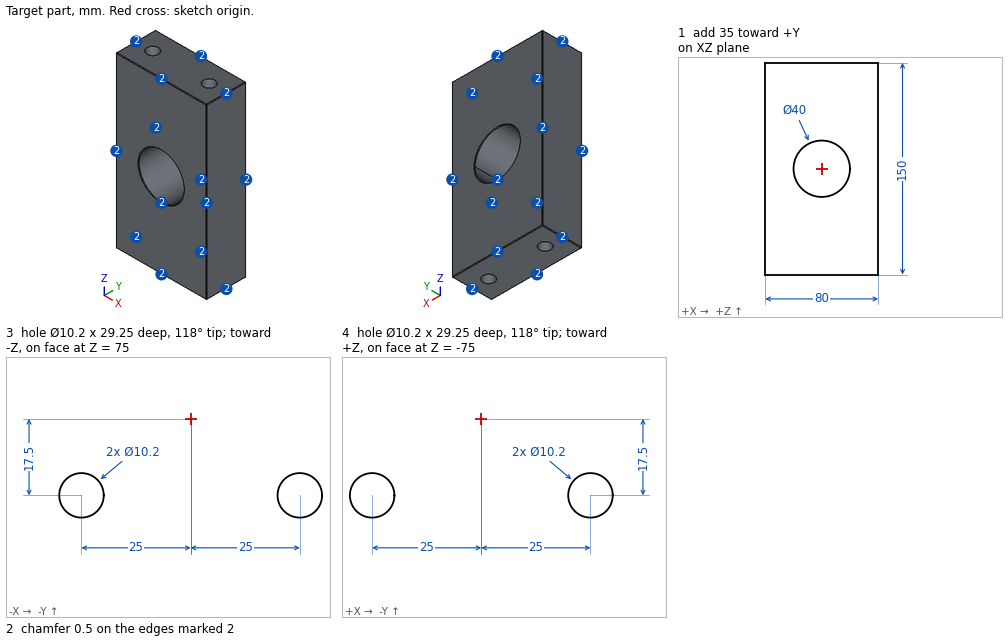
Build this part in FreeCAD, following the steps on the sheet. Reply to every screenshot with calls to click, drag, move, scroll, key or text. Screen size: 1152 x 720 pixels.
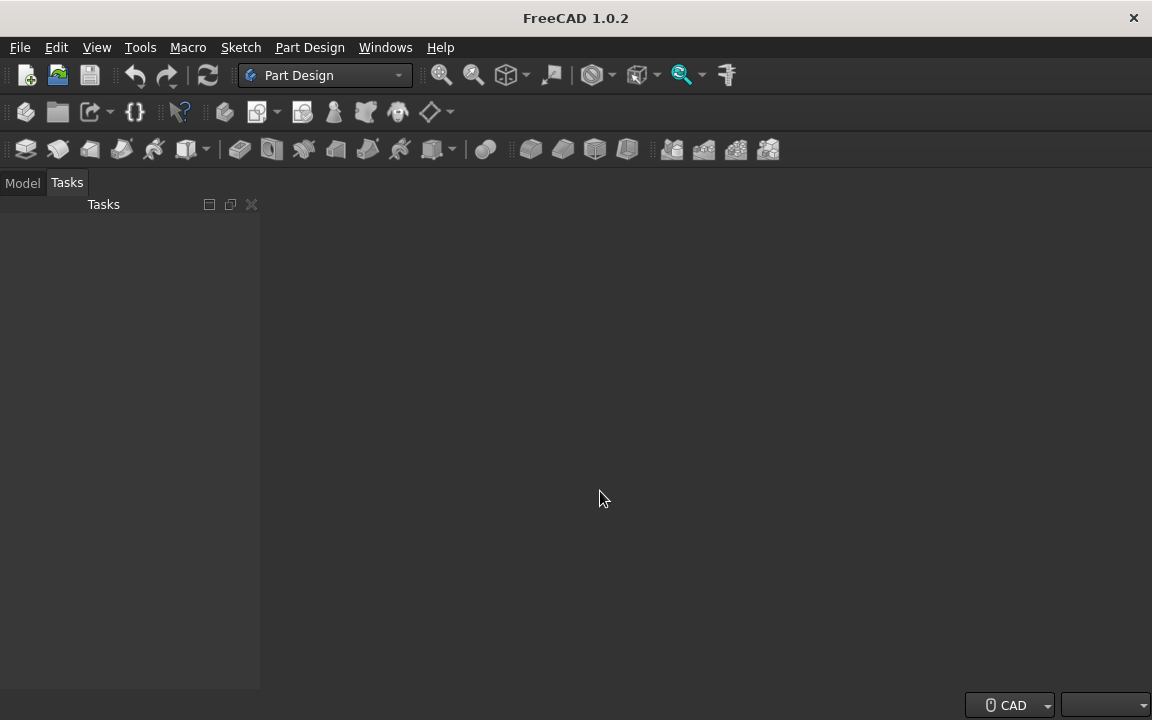
key(ctrl+n)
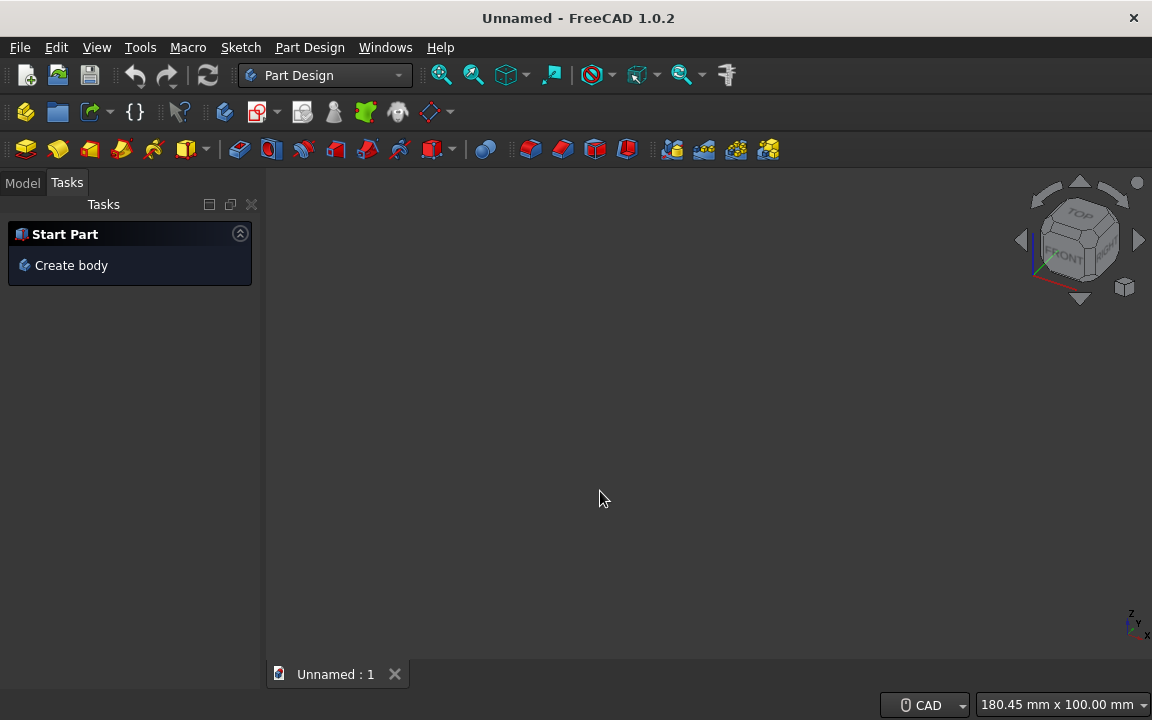
click(258, 112)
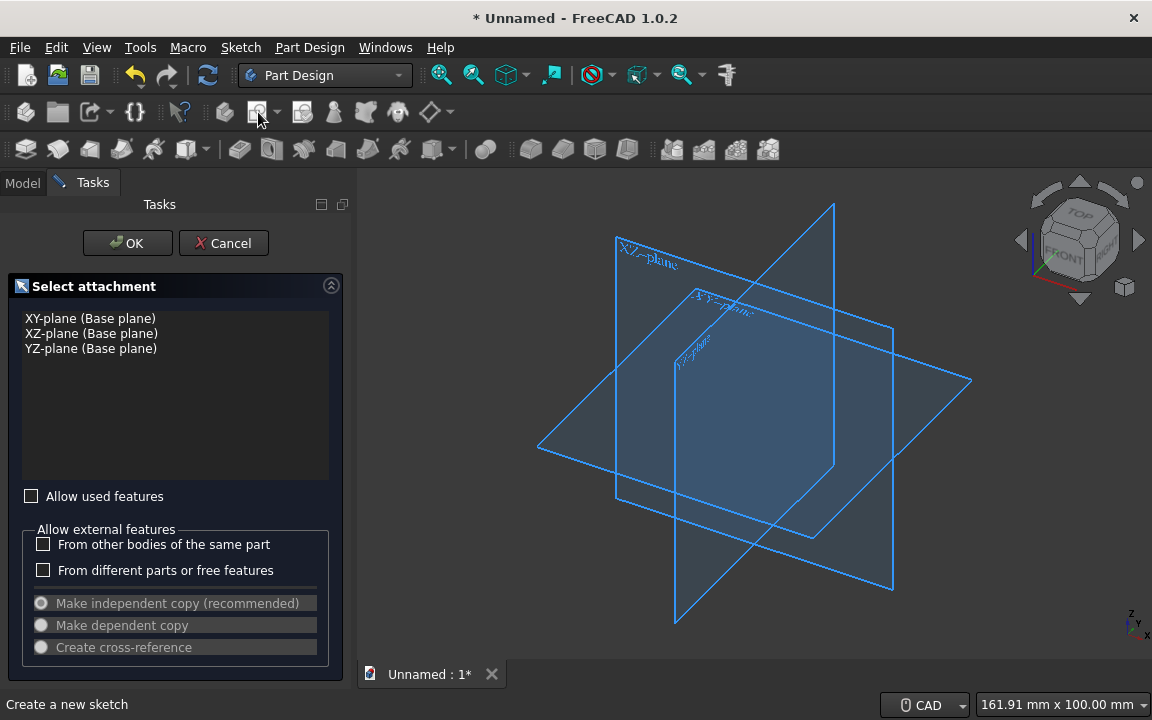
click(82, 334)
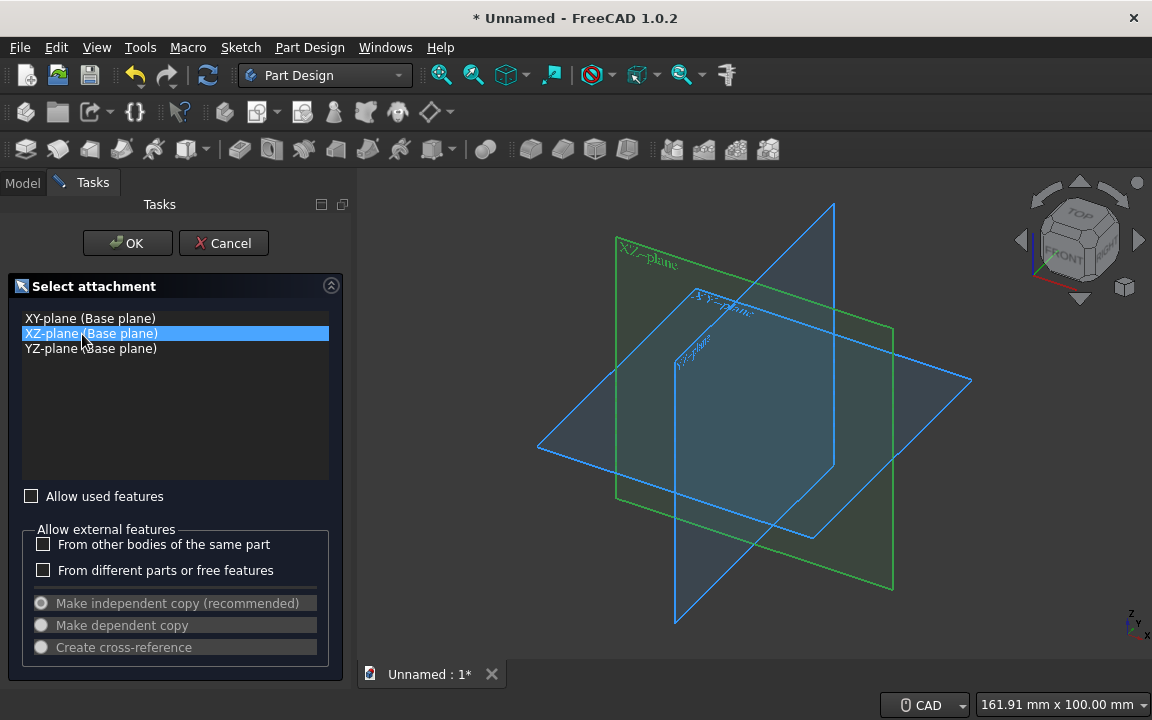
click(128, 243)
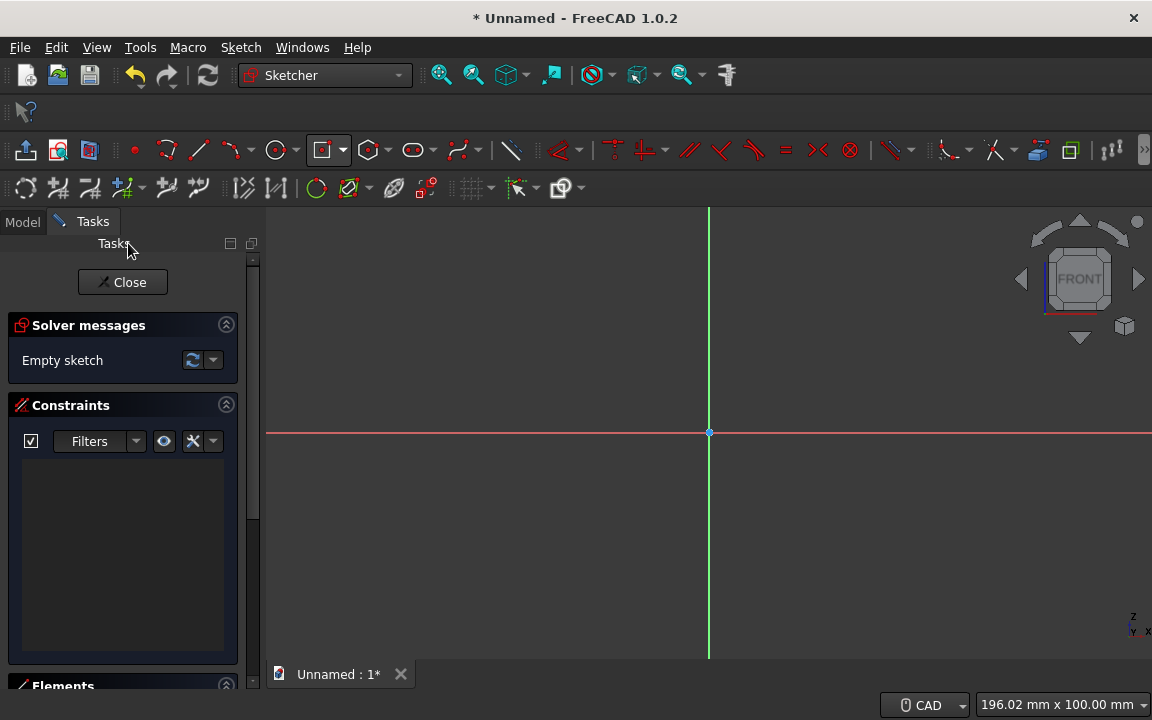
scroll(585, 433, down, 4)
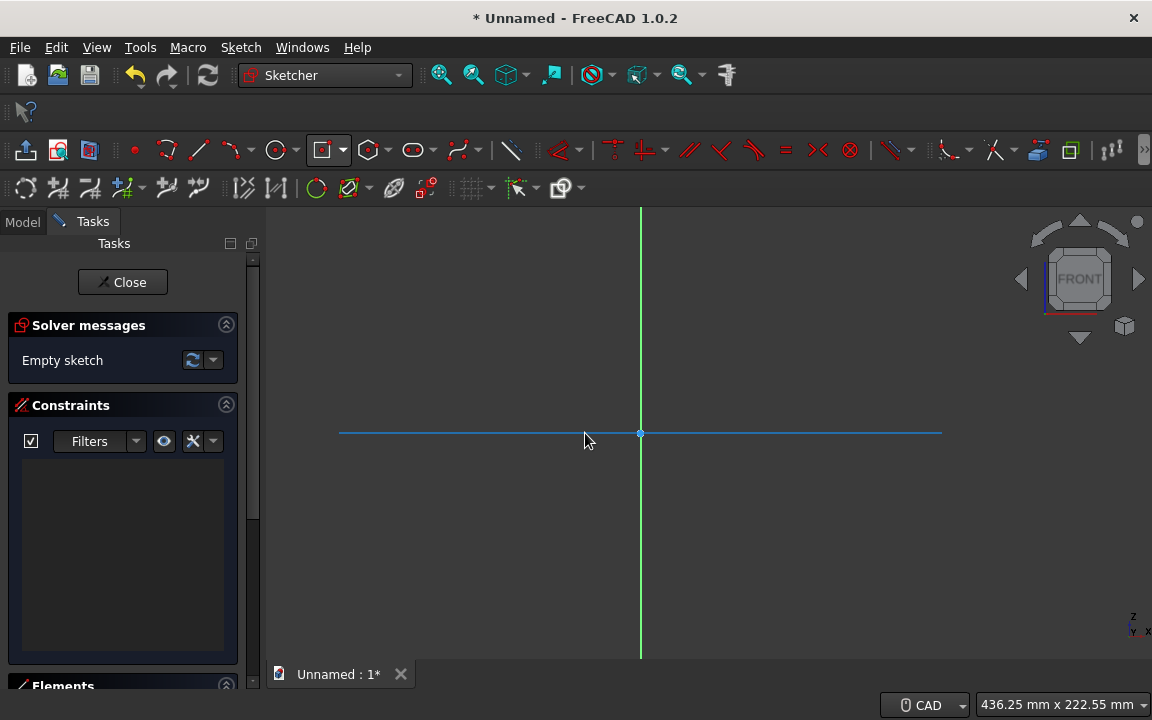
key(g)
key(v)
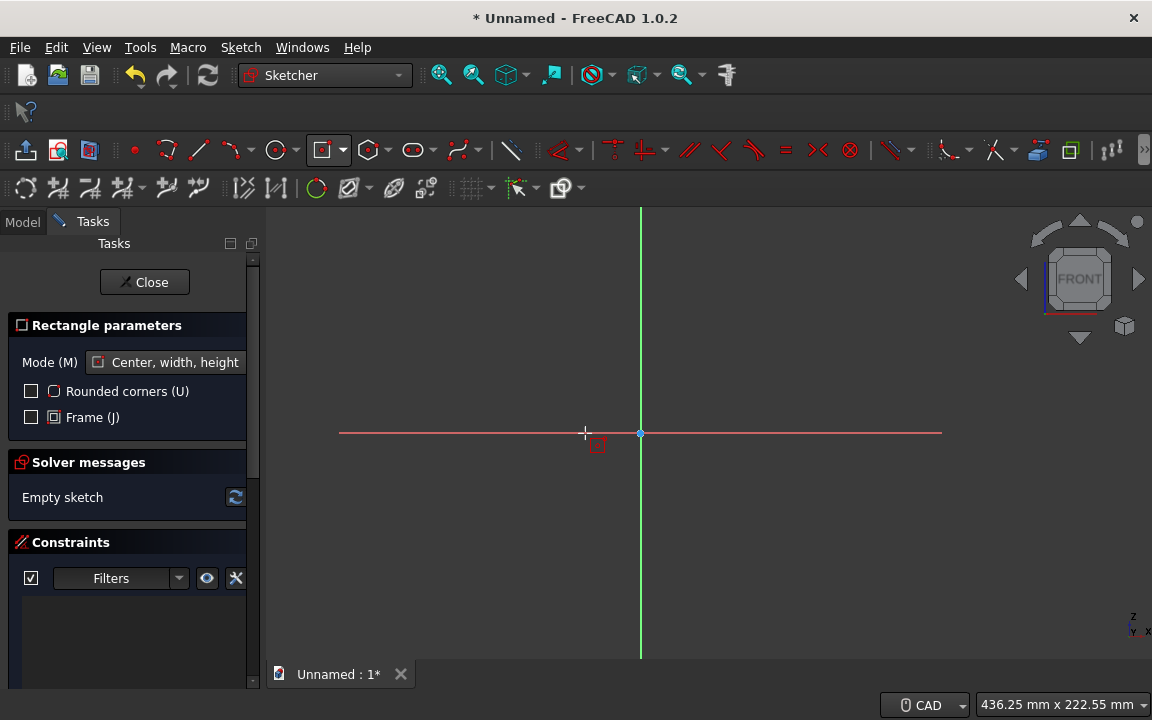
click(641, 433)
click(722, 281)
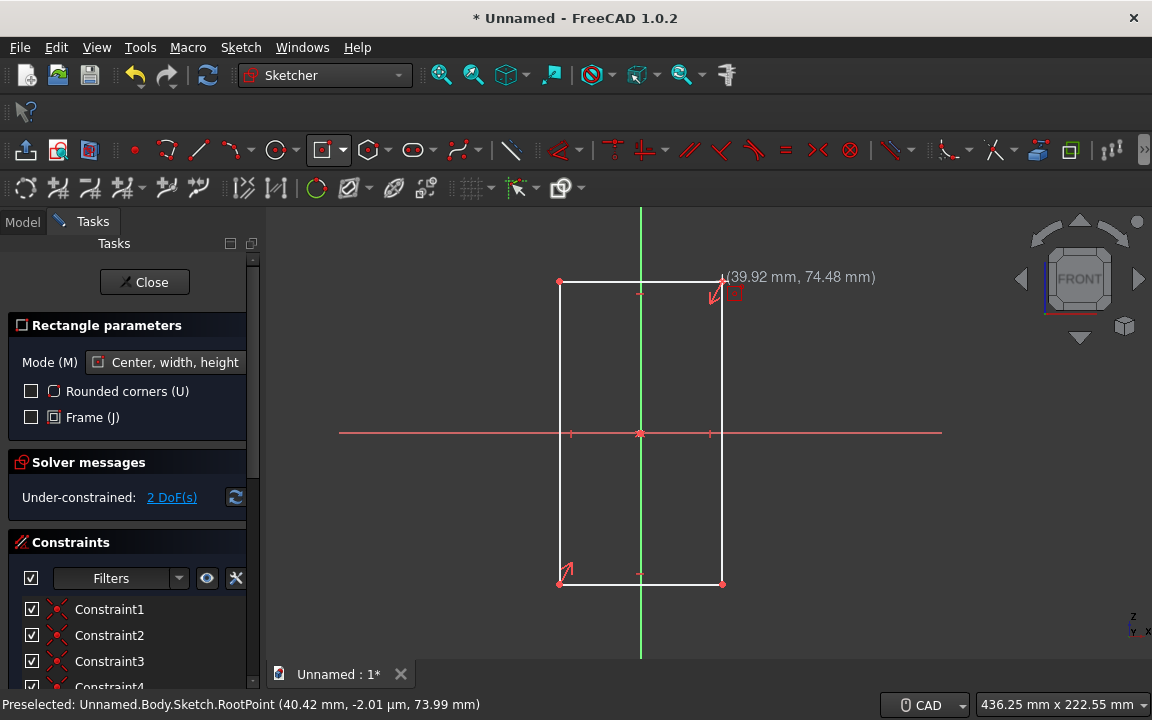
key(g)
key(c)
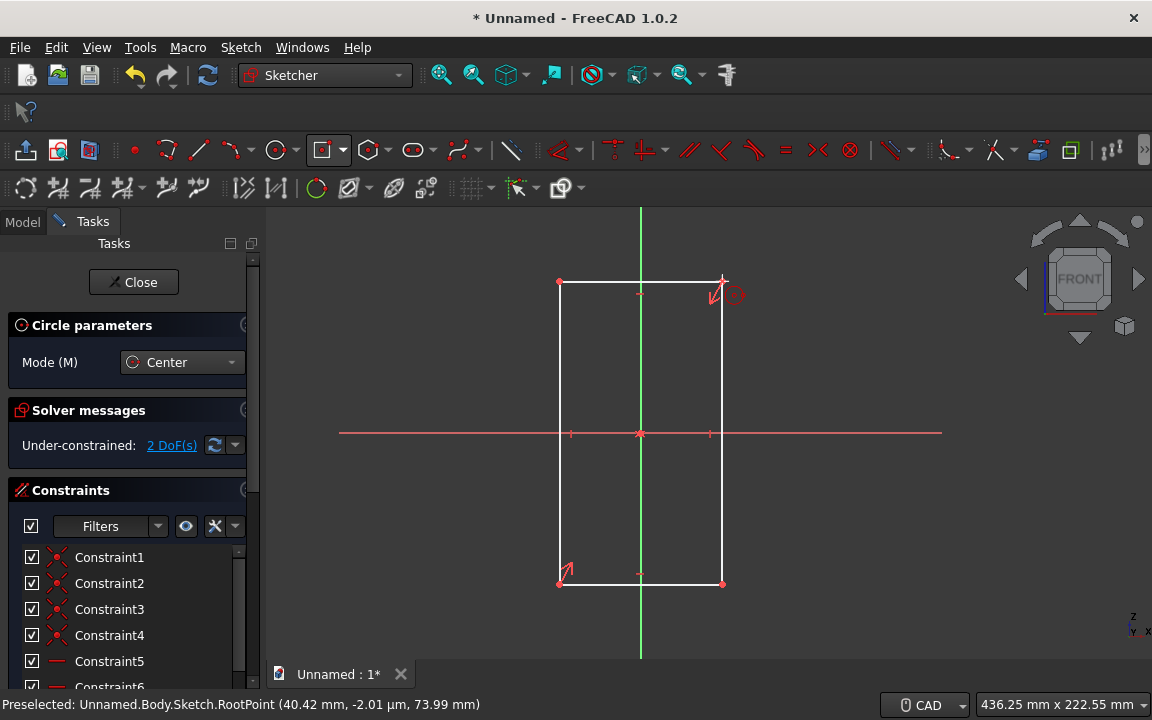
click(641, 433)
click(670, 405)
key(Escape)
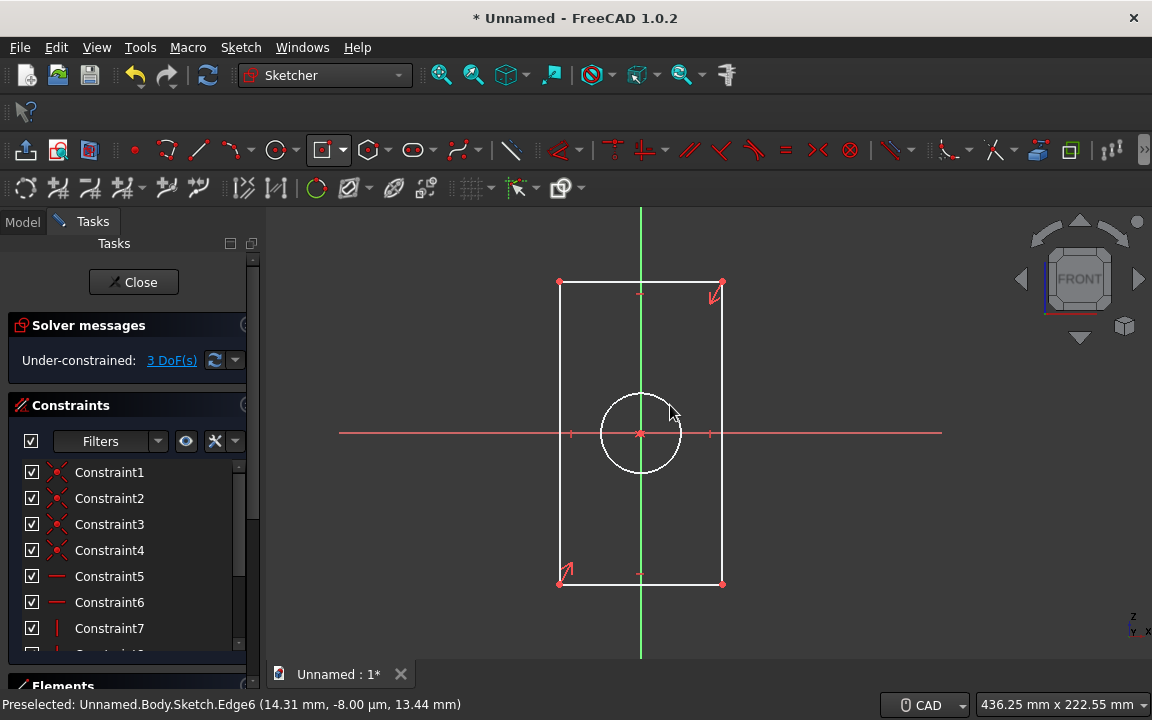
key(d)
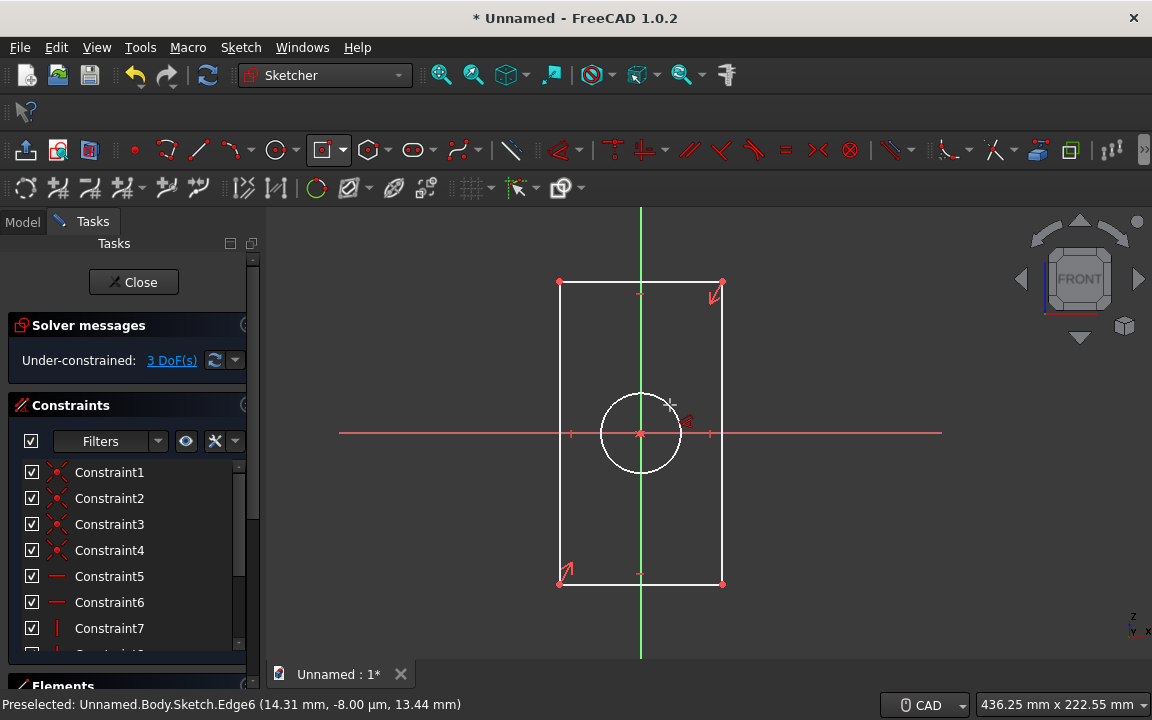
click(669, 405)
click(692, 382)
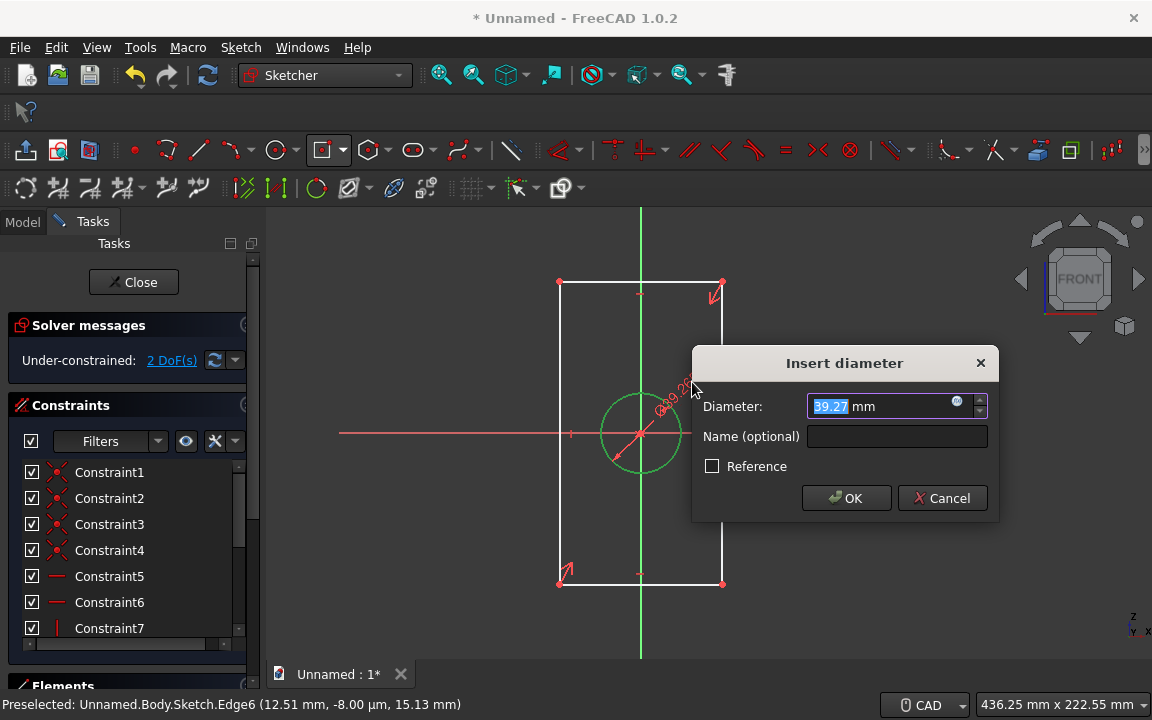
text(40)
key(Return)